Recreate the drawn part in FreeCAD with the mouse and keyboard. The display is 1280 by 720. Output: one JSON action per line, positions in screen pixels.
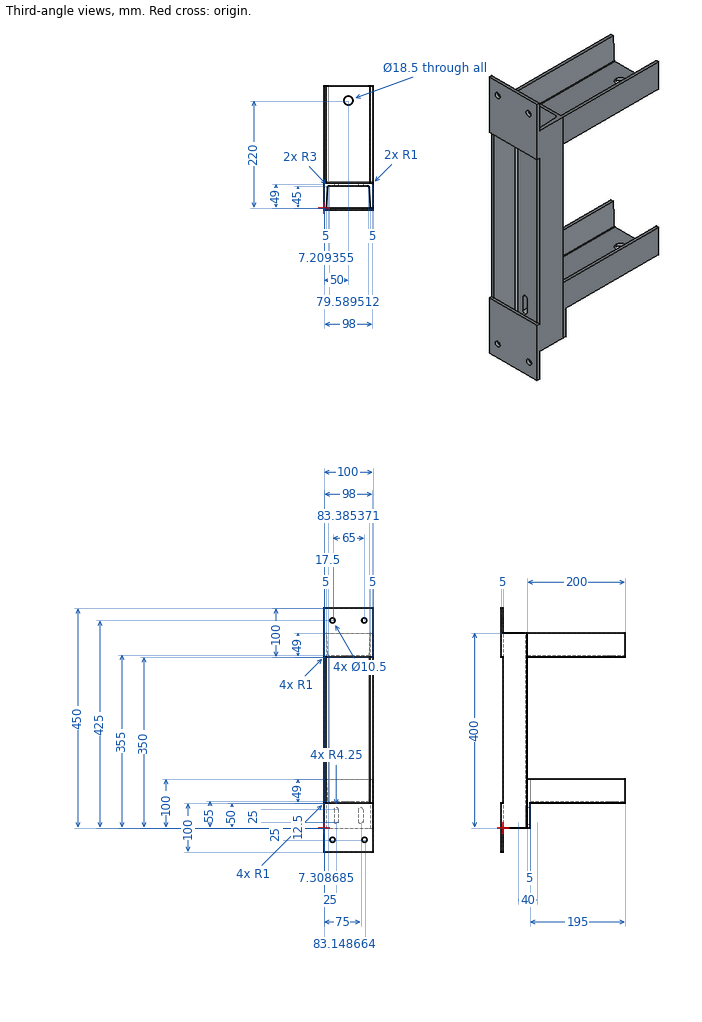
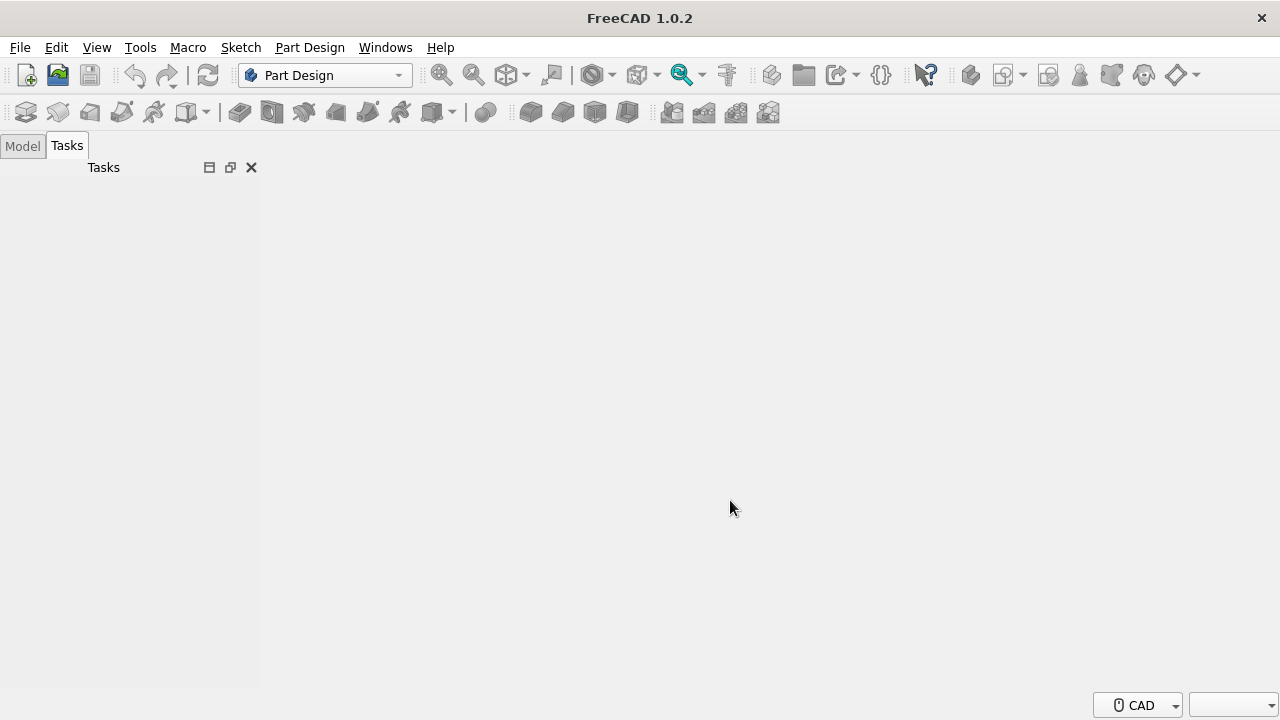
{"action": "left_click", "coordinate": [26, 76]}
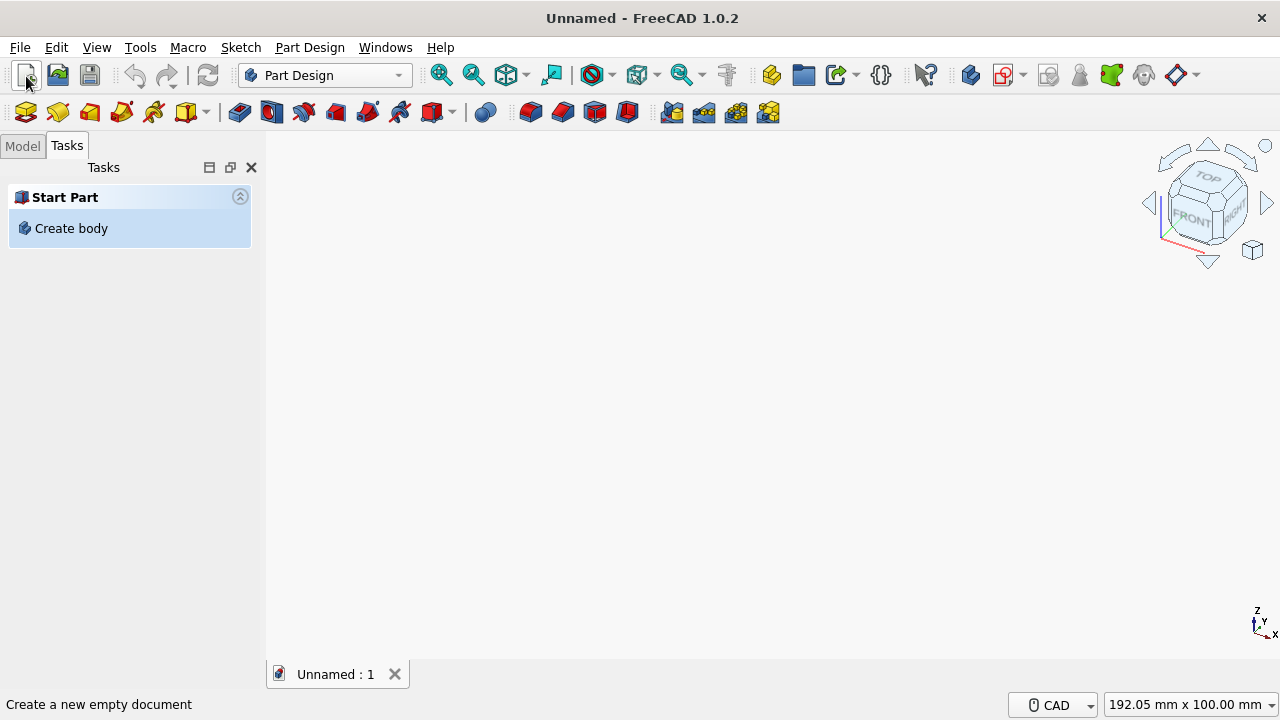
{"action": "left_click", "coordinate": [1004, 76]}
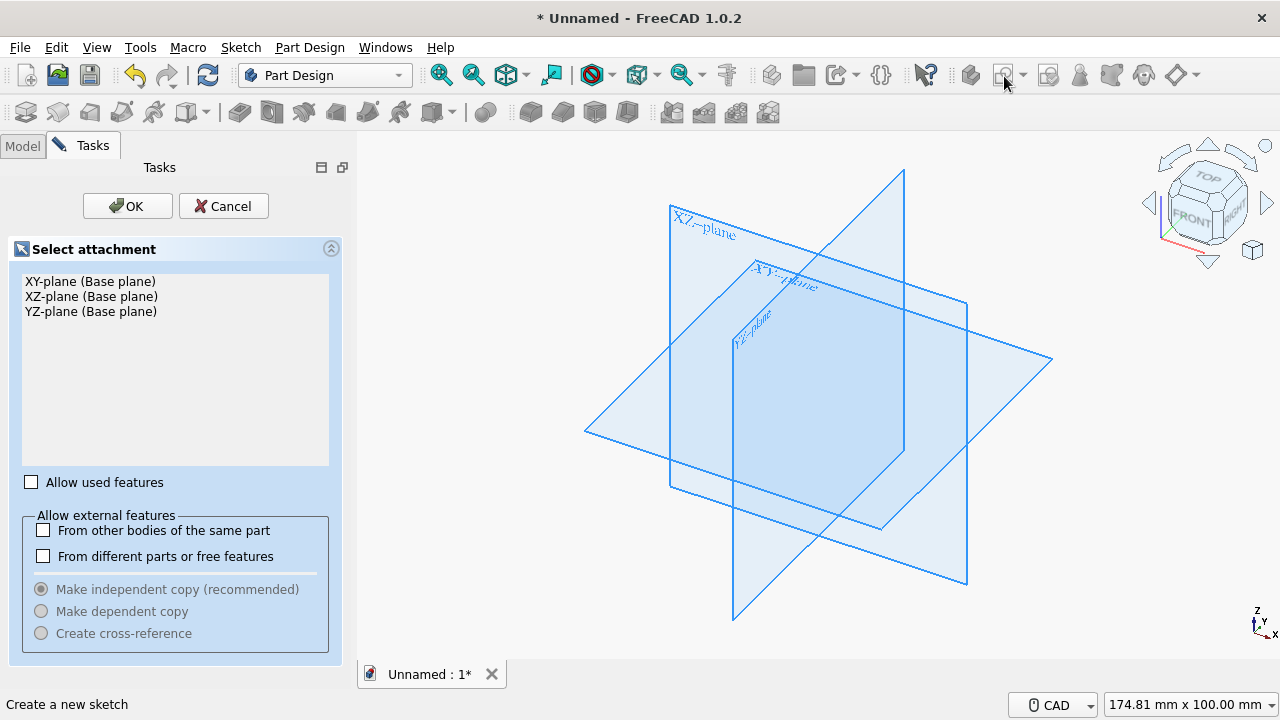
{"action": "left_click", "coordinate": [82, 282]}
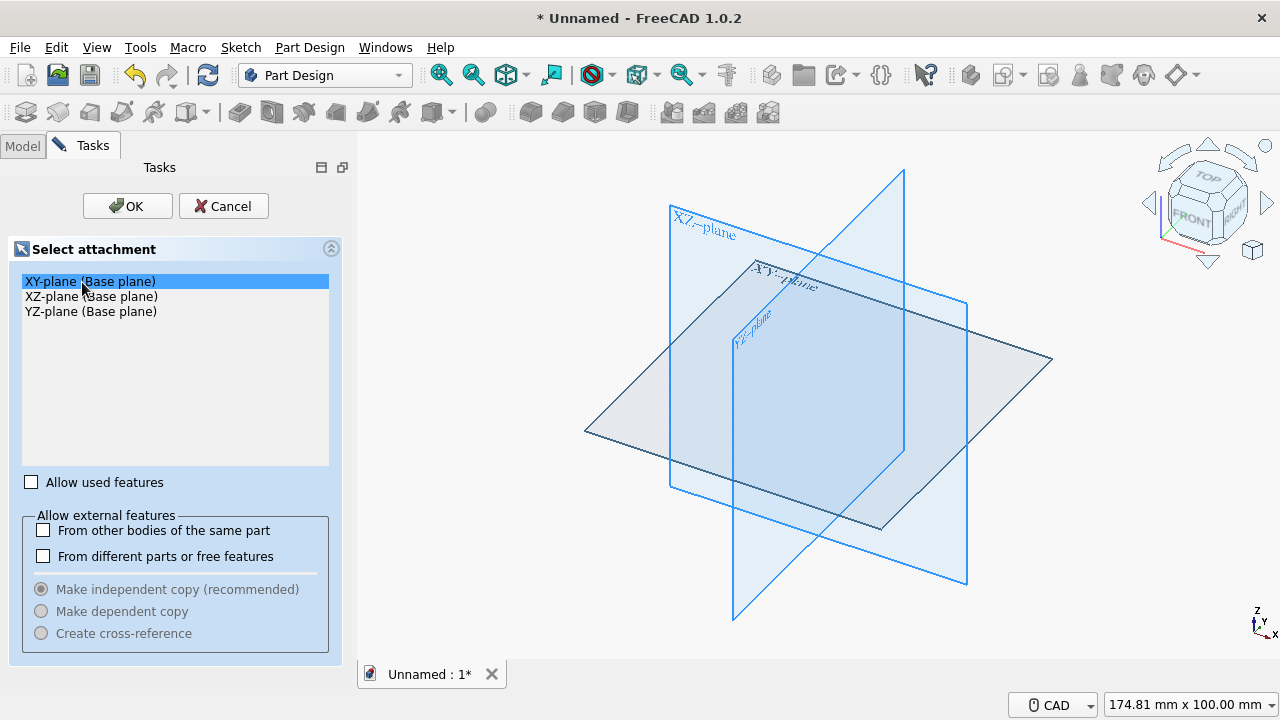
{"action": "left_click", "coordinate": [128, 206]}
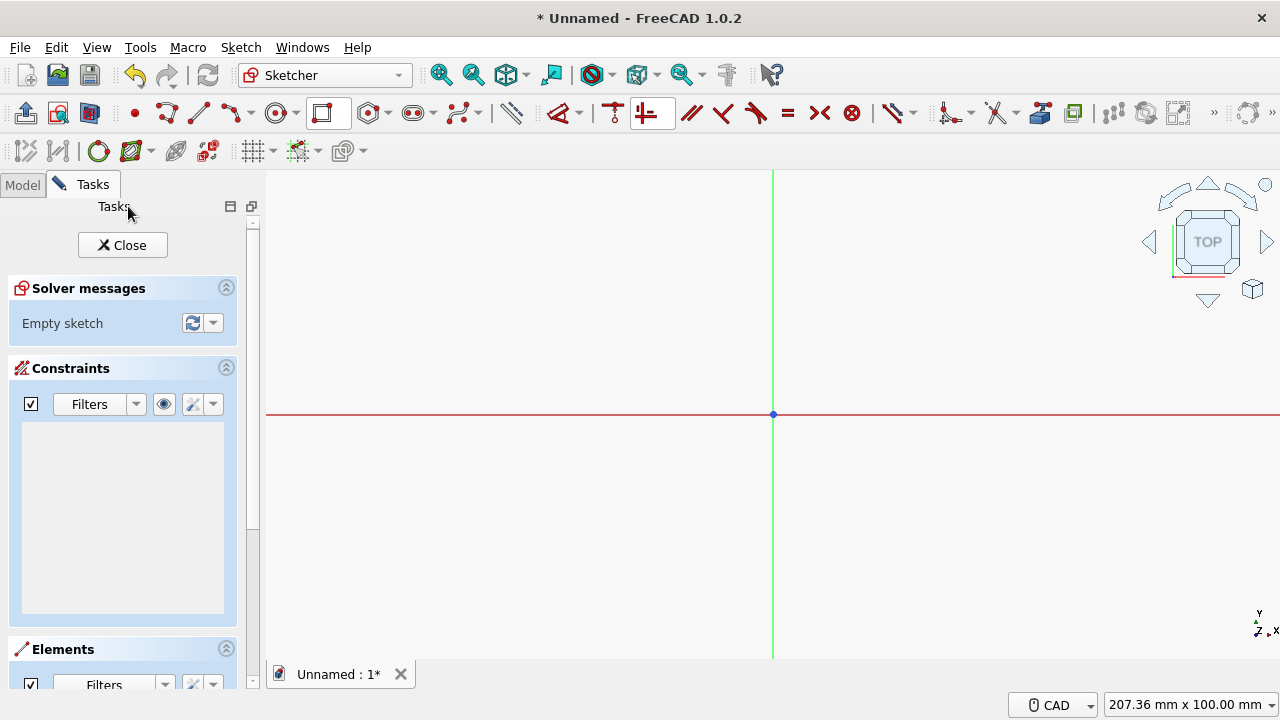
{"action": "scroll", "coordinate": [294, 631], "scroll_direction": "down", "scroll_amount": 1}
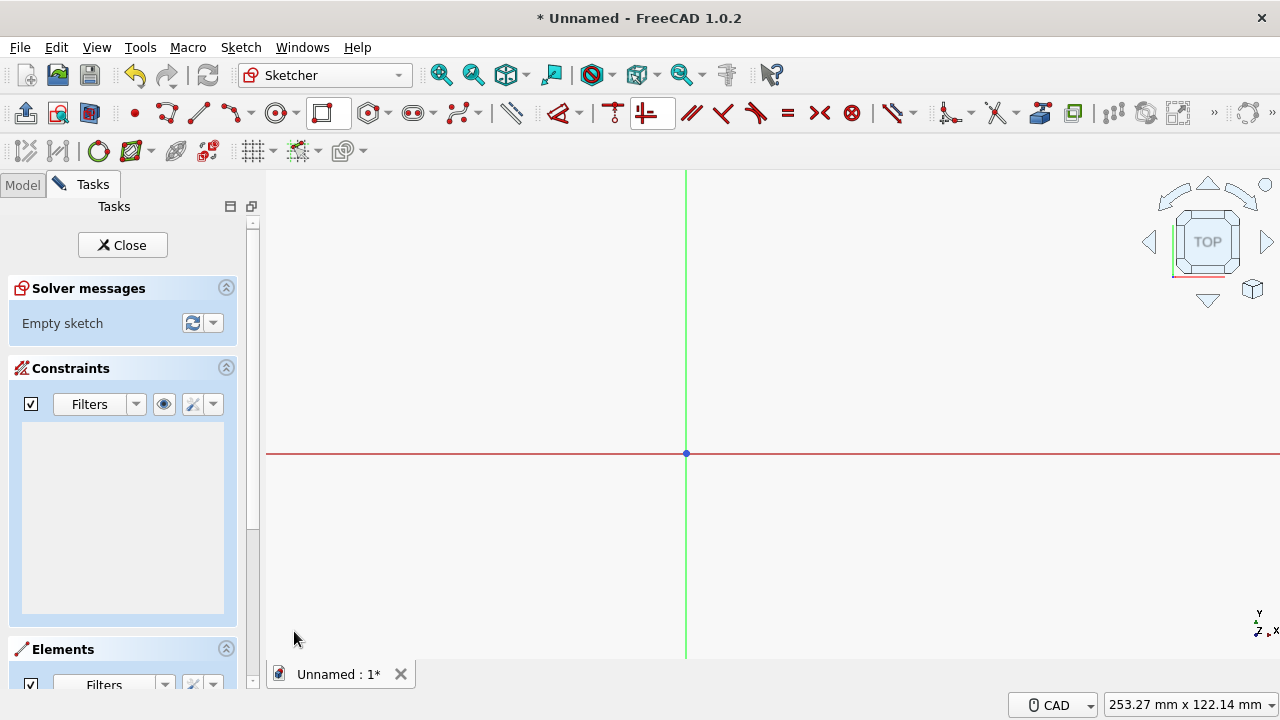
{"action": "scroll", "coordinate": [1115, 230], "scroll_direction": "up", "scroll_amount": 2}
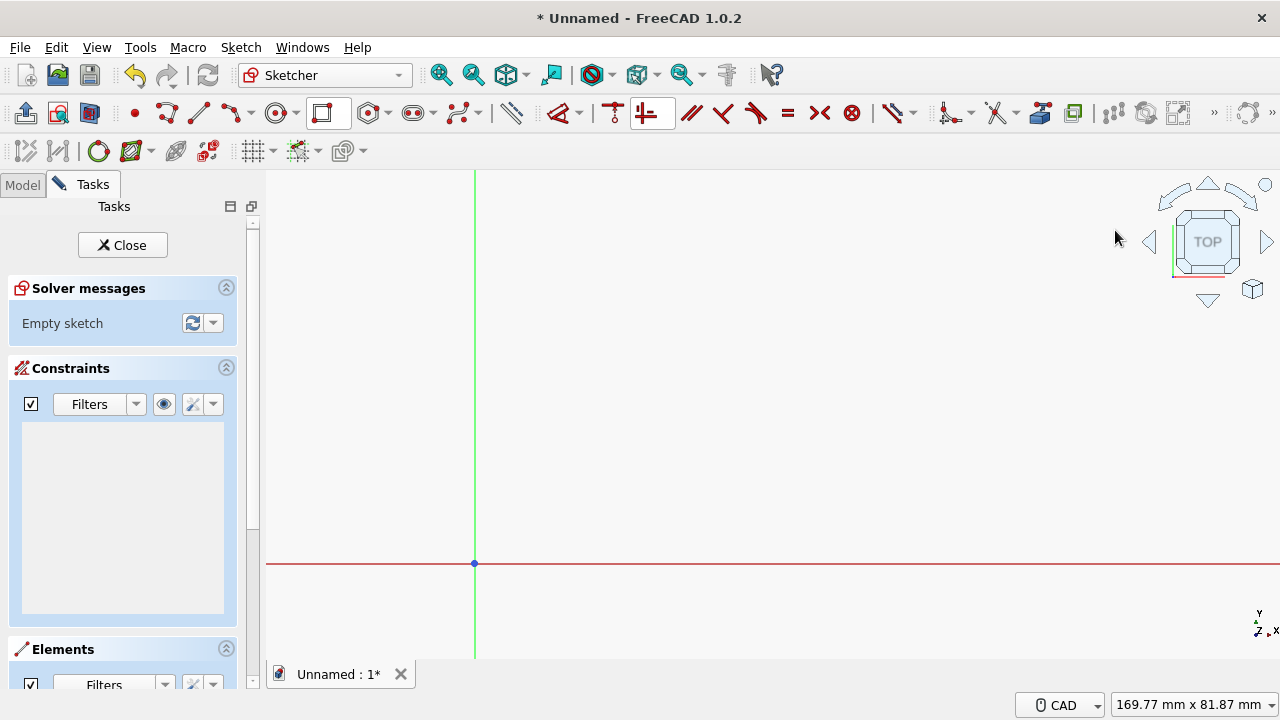
{"action": "left_click", "coordinate": [168, 114]}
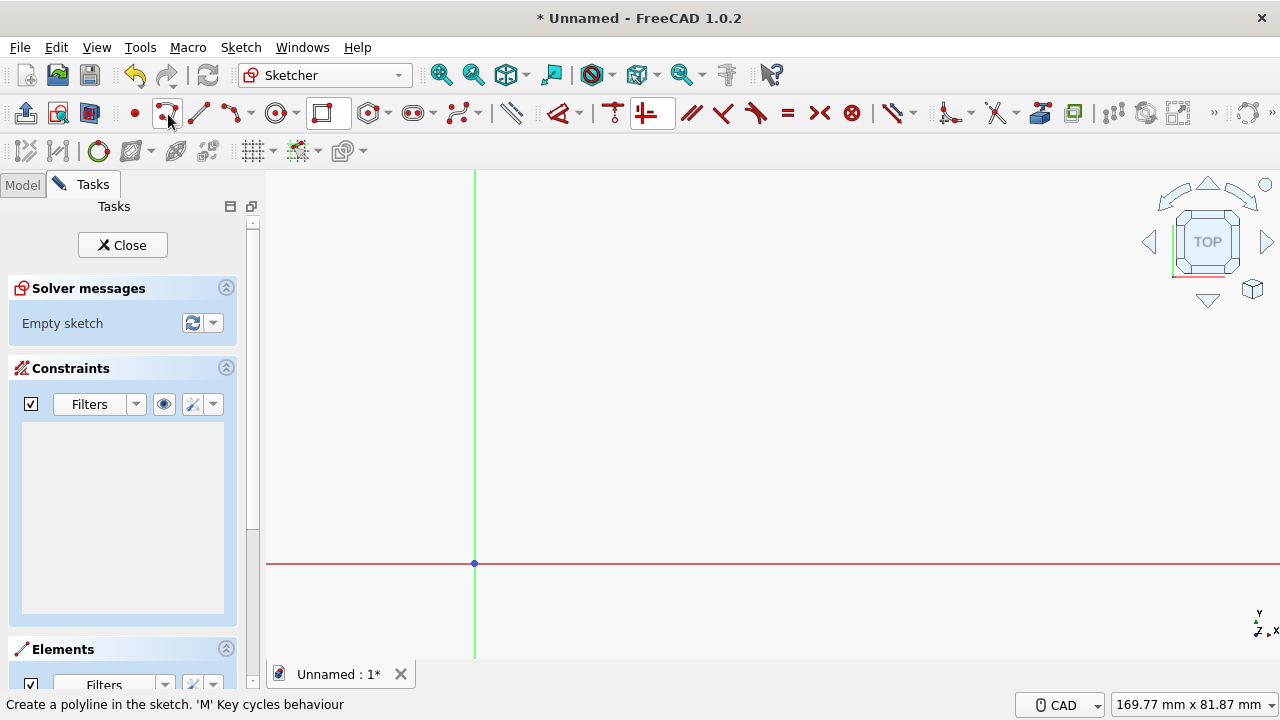
{"action": "left_click", "coordinate": [475, 271]}
{"action": "left_click", "coordinate": [475, 564]}
{"action": "left_click", "coordinate": [505, 555]}
{"action": "left_click", "coordinate": [518, 312]}
{"action": "right_click", "coordinate": [518, 312]}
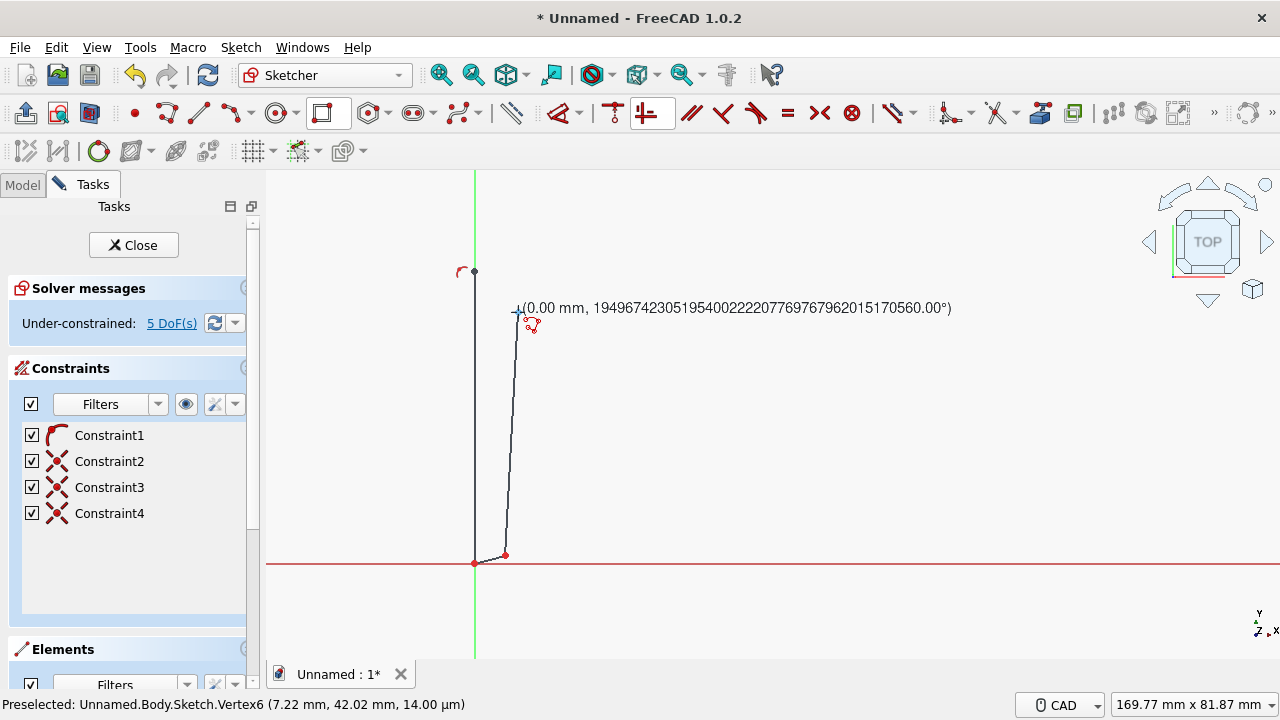
{"action": "key", "text": "g l"}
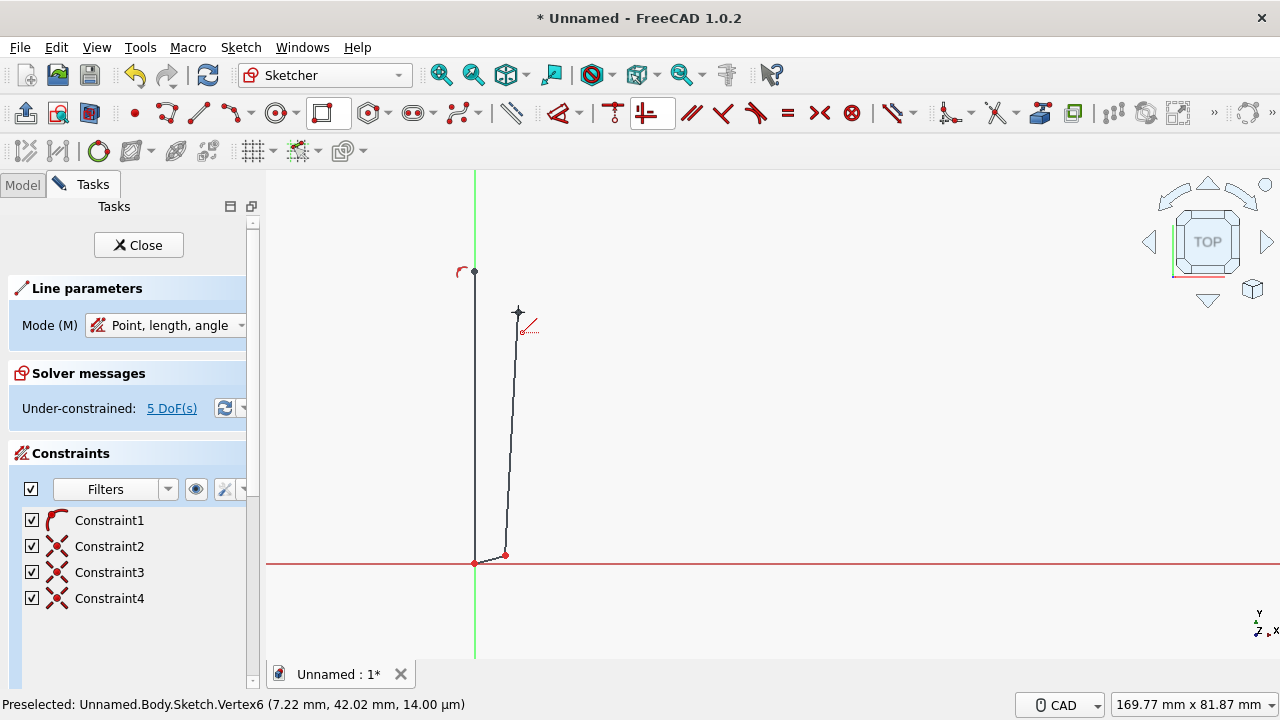
{"action": "left_click", "coordinate": [536, 295]}
{"action": "left_click", "coordinate": [1011, 295]}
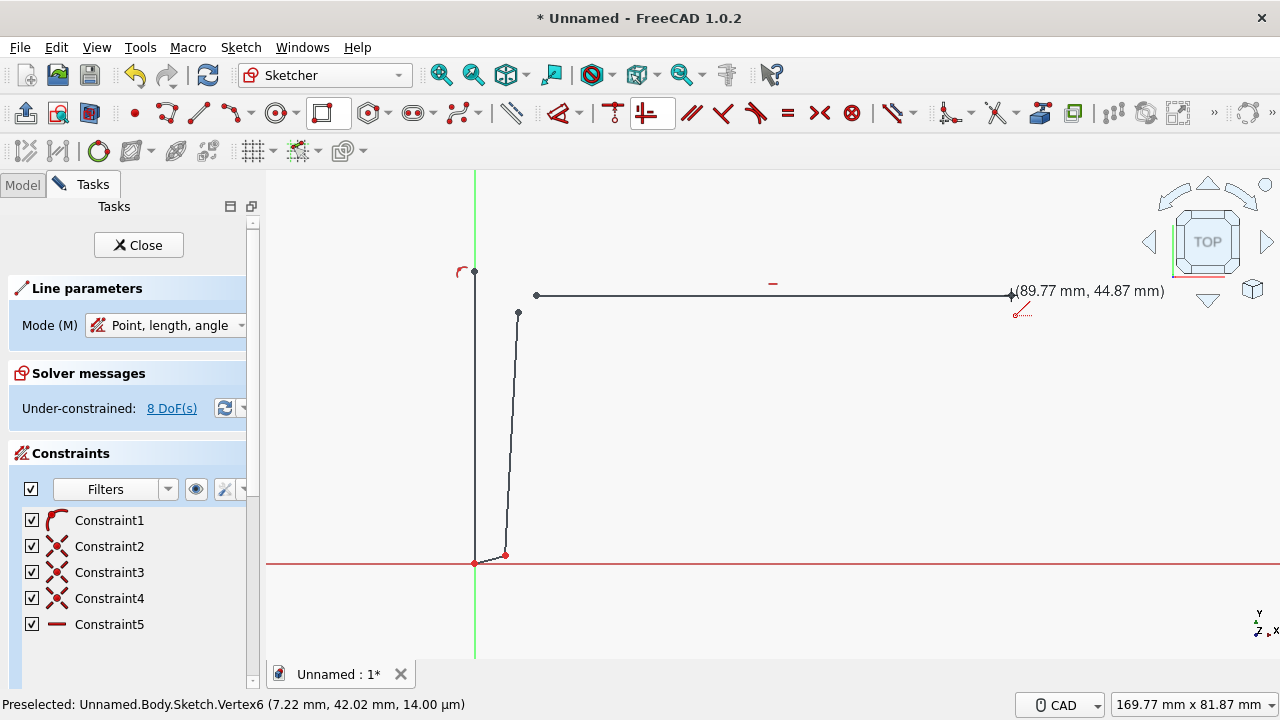
{"action": "left_click", "coordinate": [168, 114]}